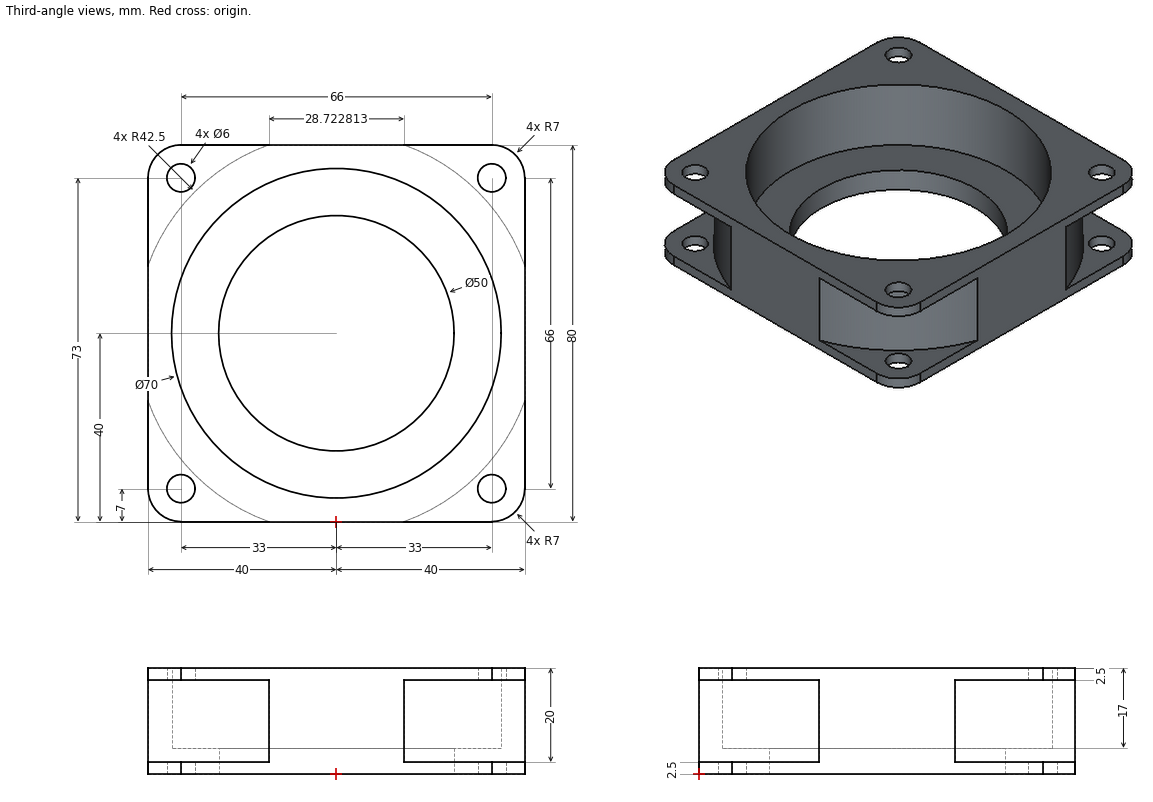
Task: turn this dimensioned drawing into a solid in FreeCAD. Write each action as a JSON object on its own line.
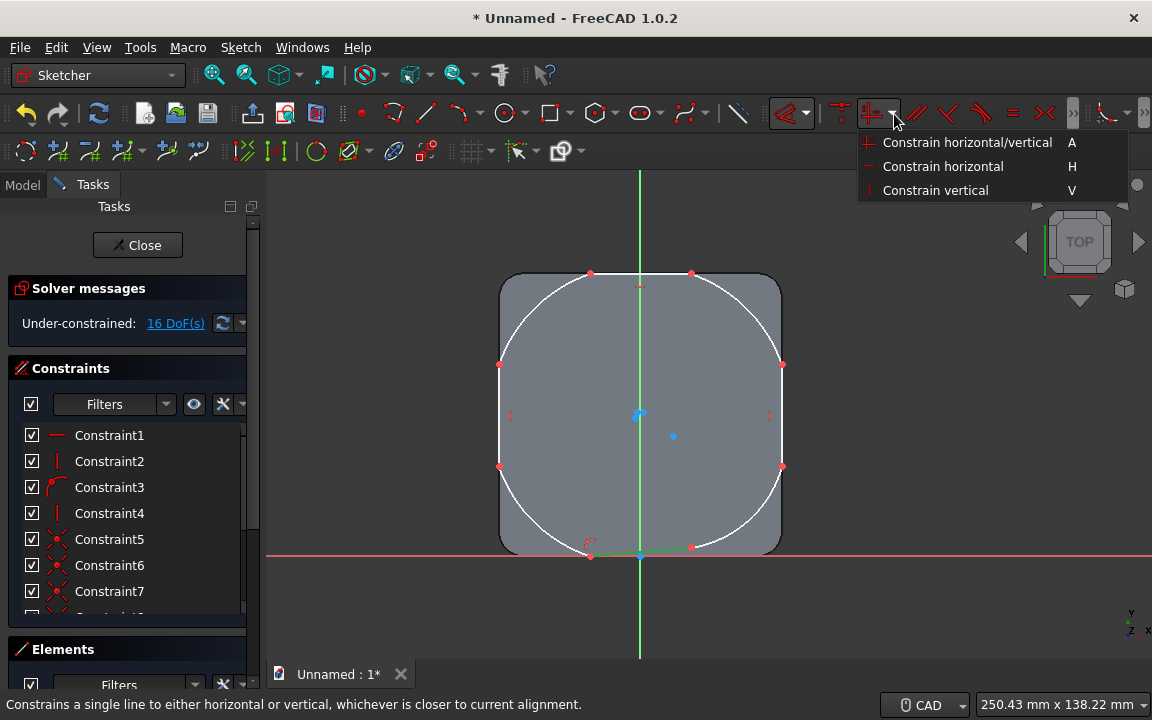
{"action": "left_click", "coordinate": [993, 166]}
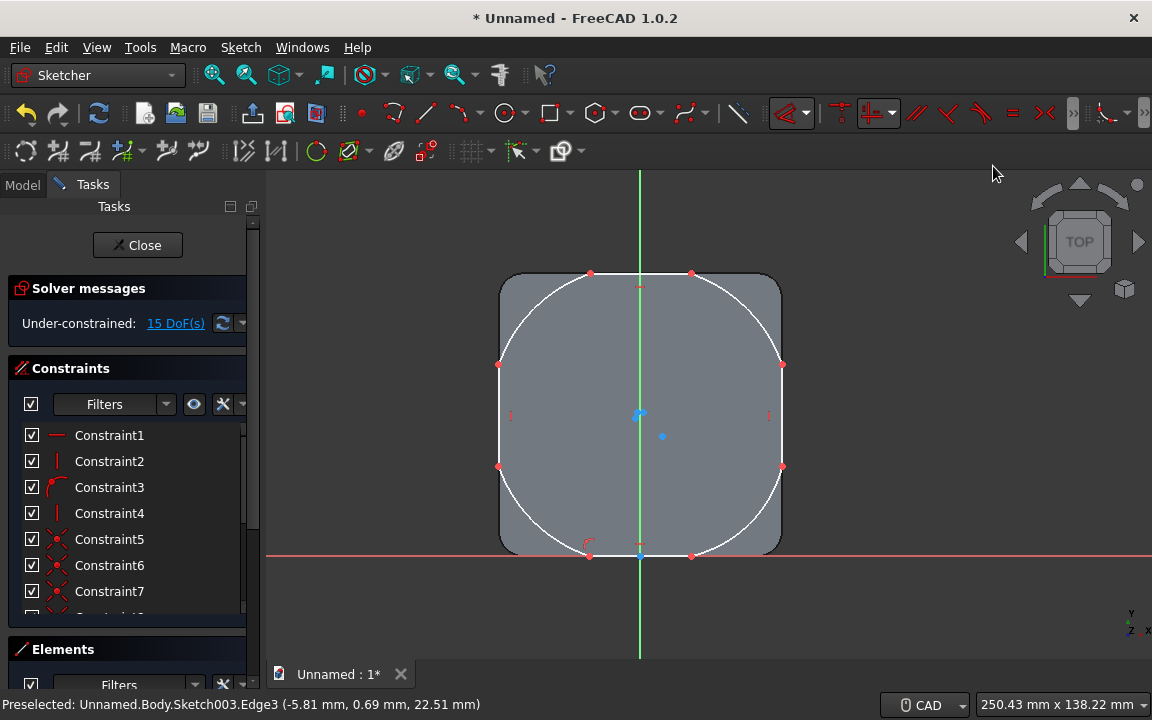
{"action": "left_click", "coordinate": [554, 292]}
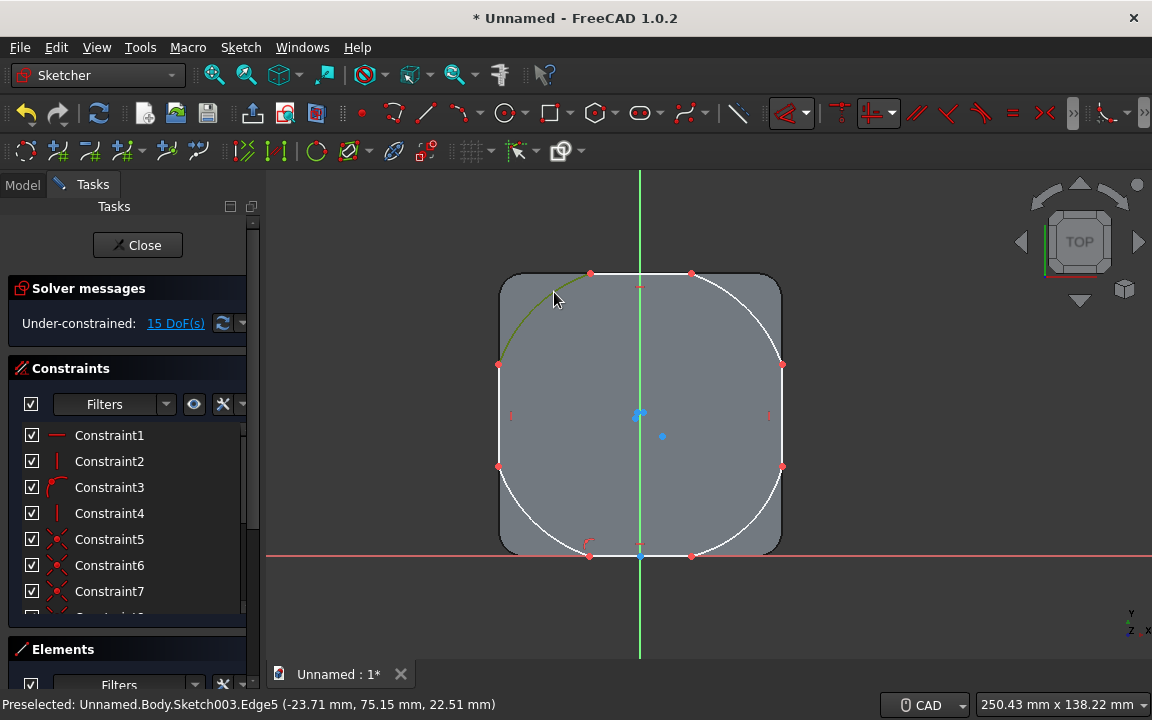
{"action": "left_click", "coordinate": [517, 502]}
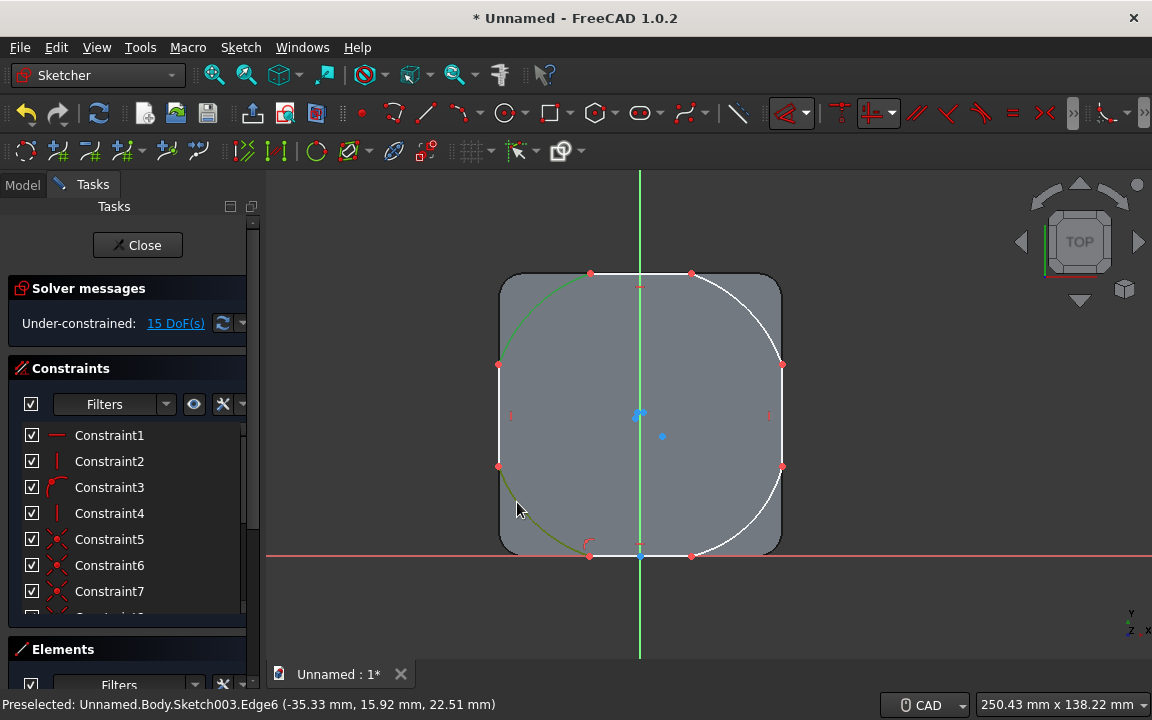
{"action": "left_click", "coordinate": [840, 114]}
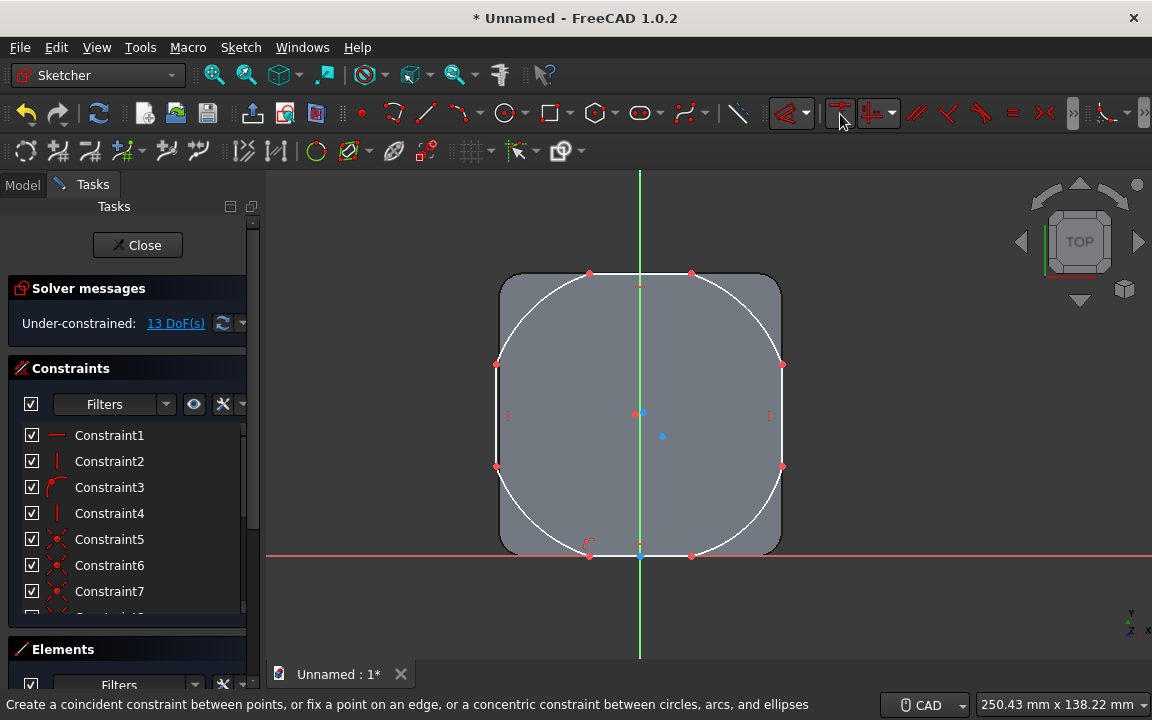
{"action": "left_click", "coordinate": [554, 292]}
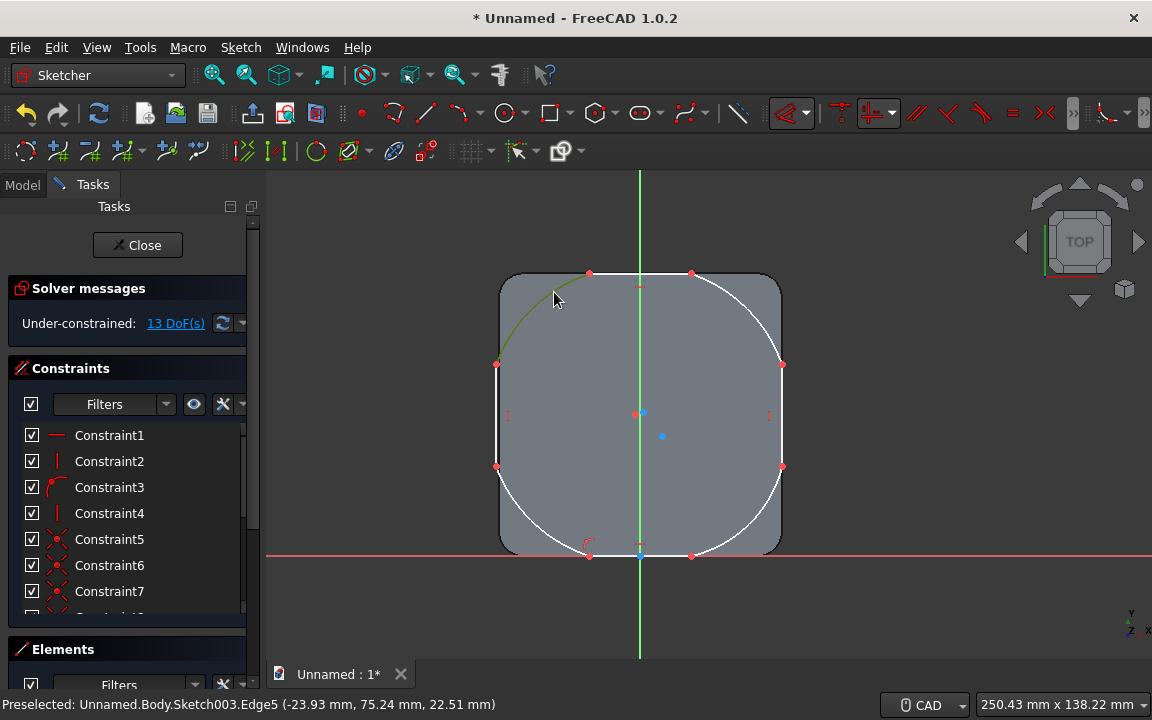
{"action": "left_click", "coordinate": [728, 541]}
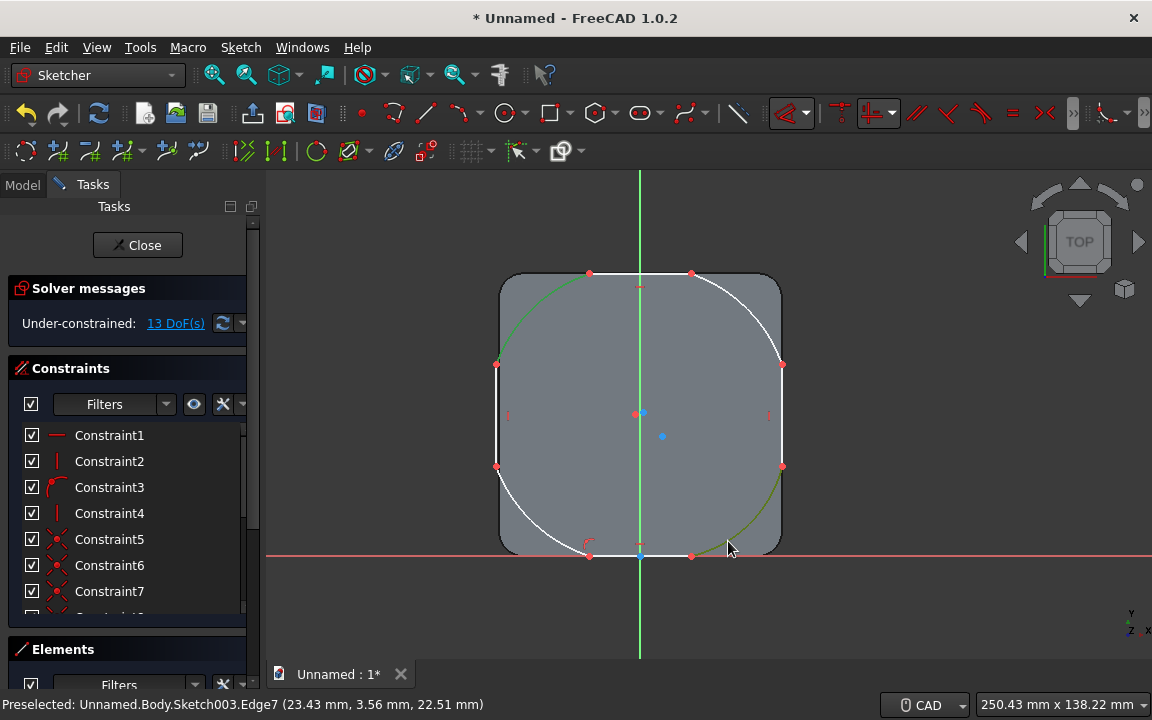
{"action": "key", "text": "c"}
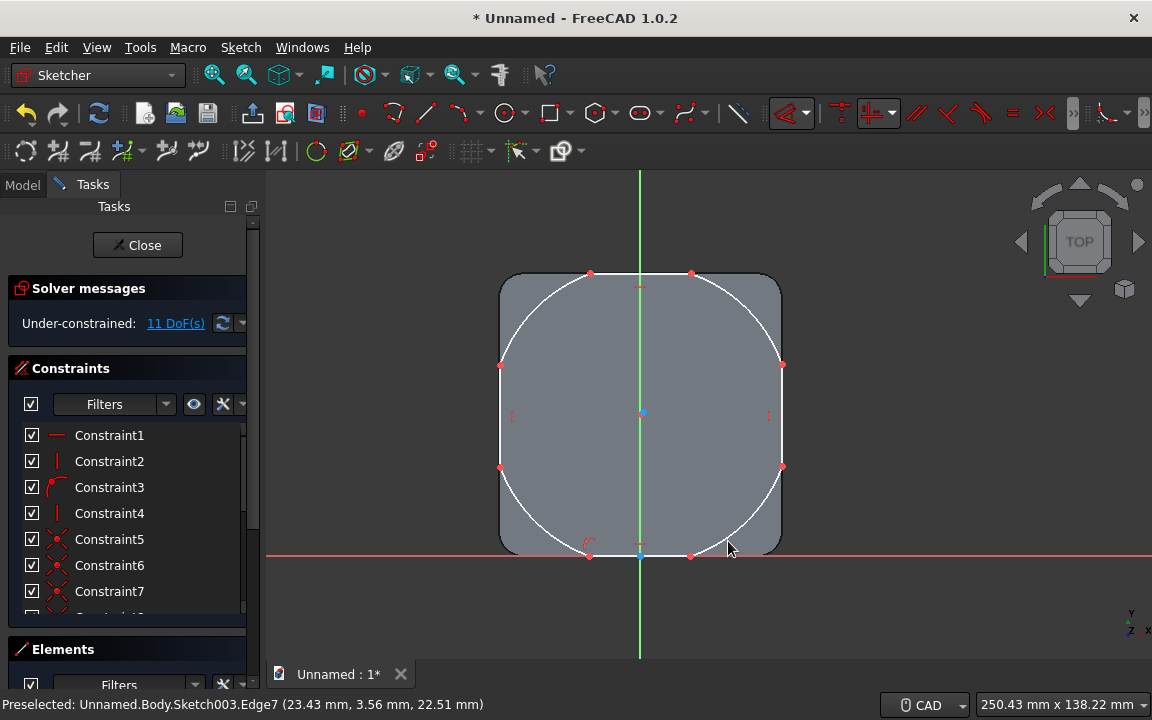
{"action": "left_click", "coordinate": [555, 292]}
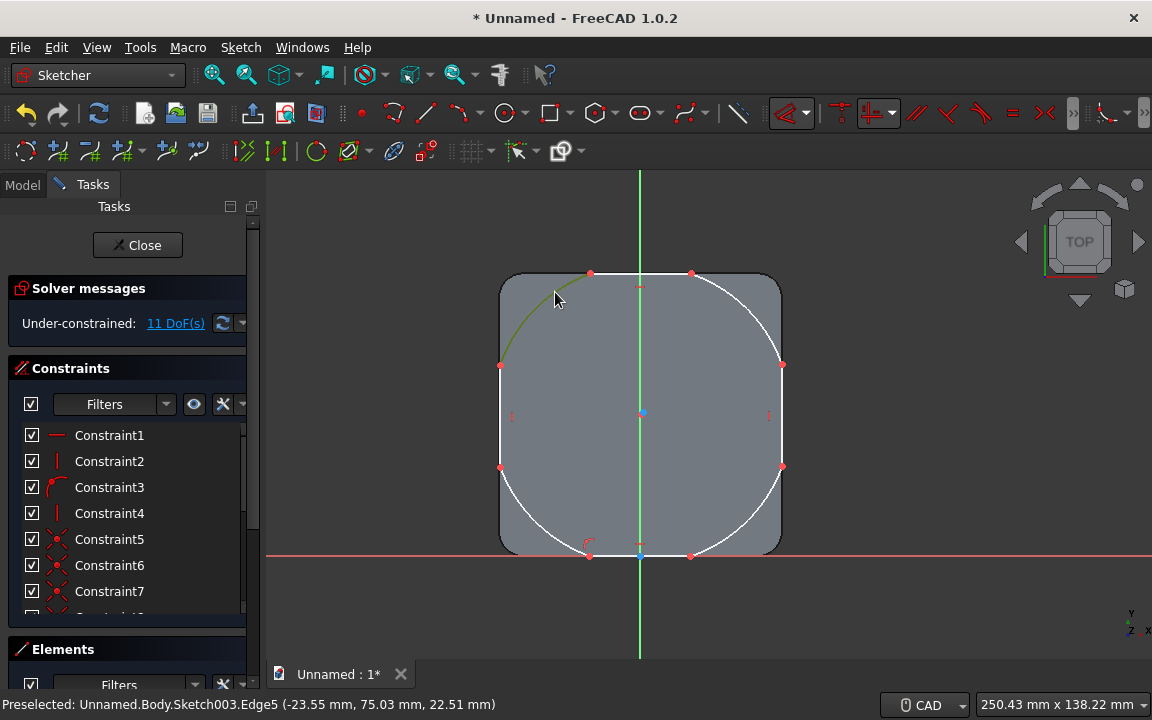
{"action": "left_click", "coordinate": [764, 329]}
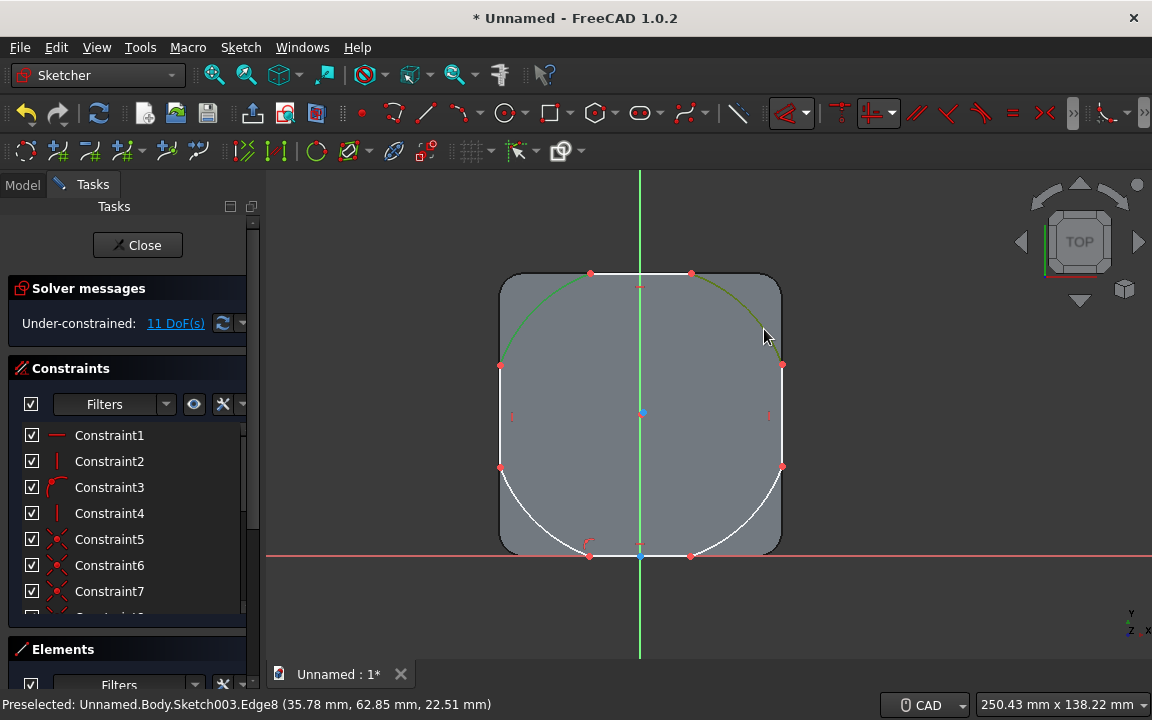
{"action": "key", "text": "c"}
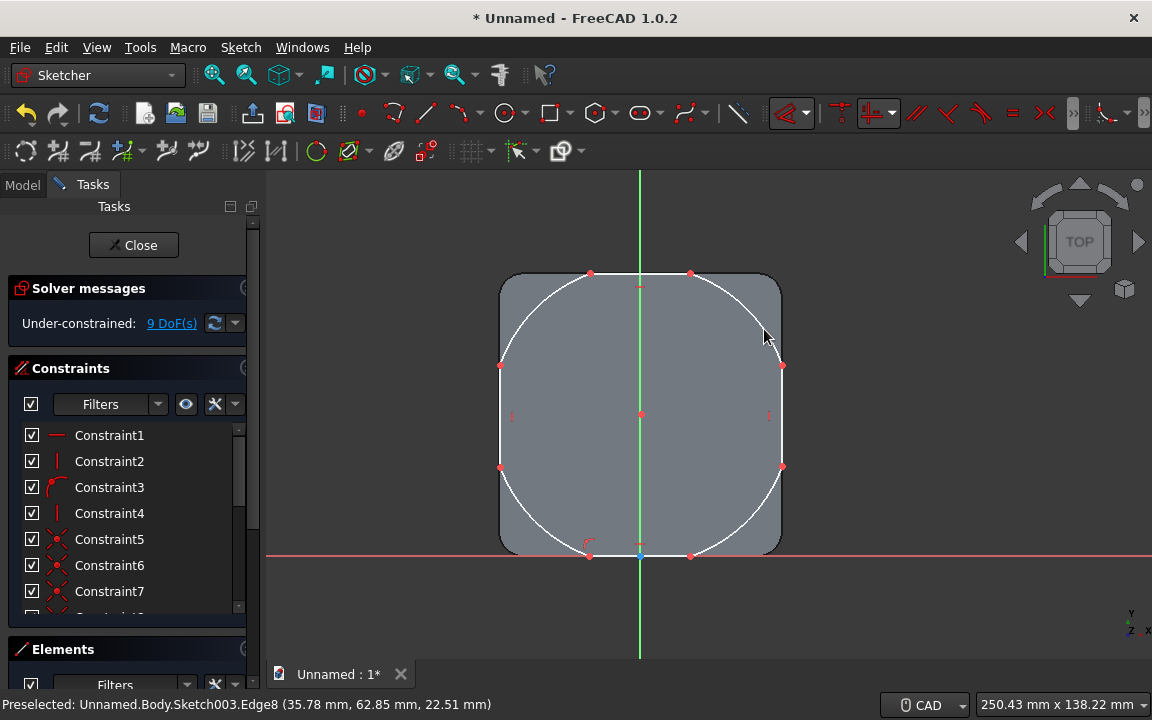
{"action": "left_click", "coordinate": [555, 292]}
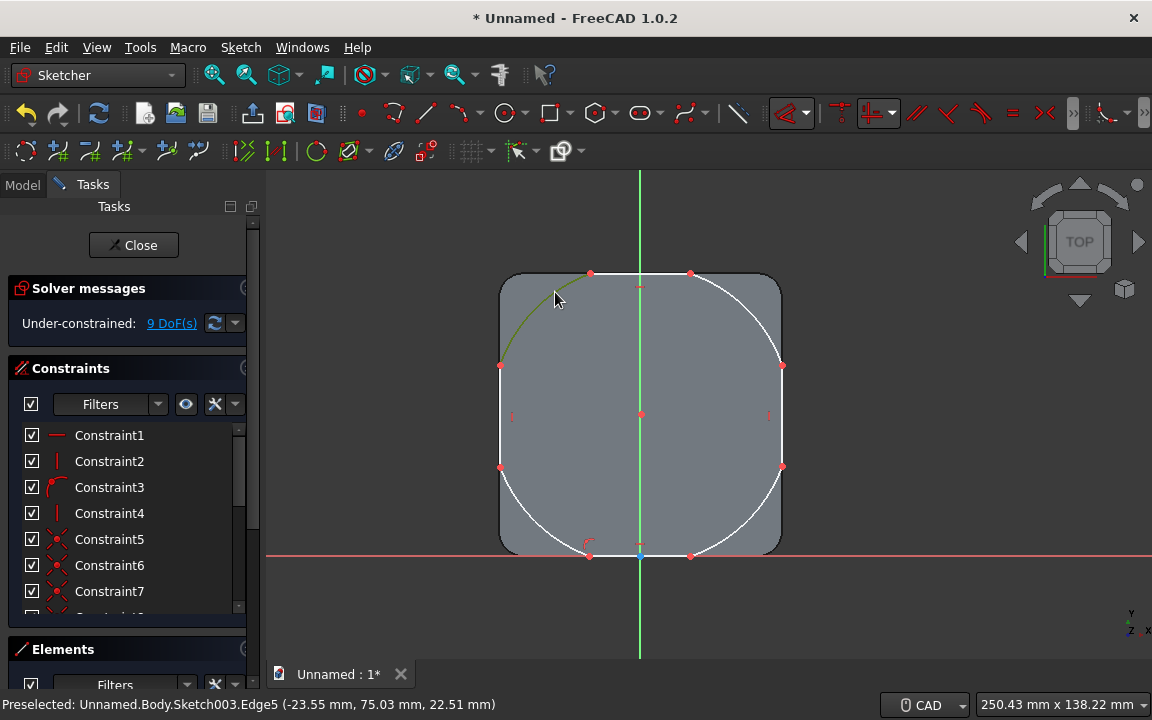
{"action": "left_click", "coordinate": [518, 502]}